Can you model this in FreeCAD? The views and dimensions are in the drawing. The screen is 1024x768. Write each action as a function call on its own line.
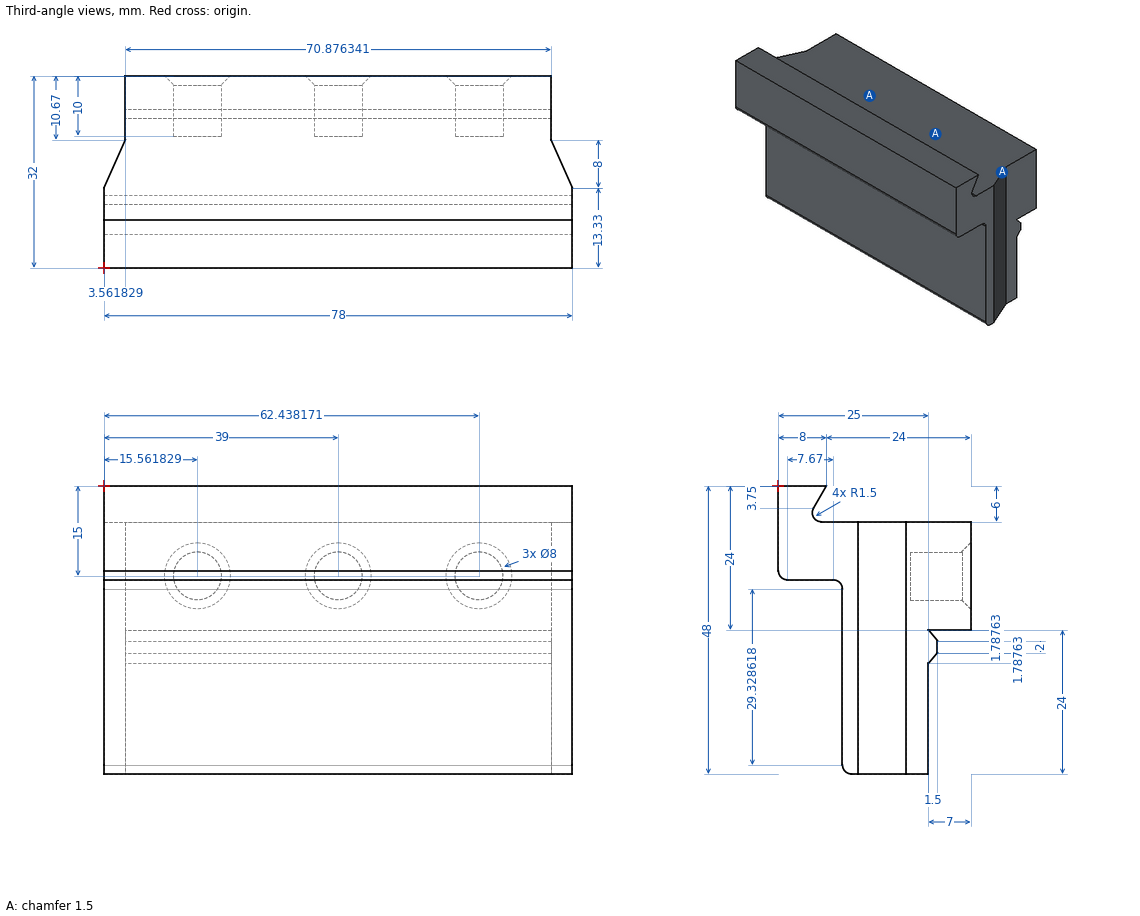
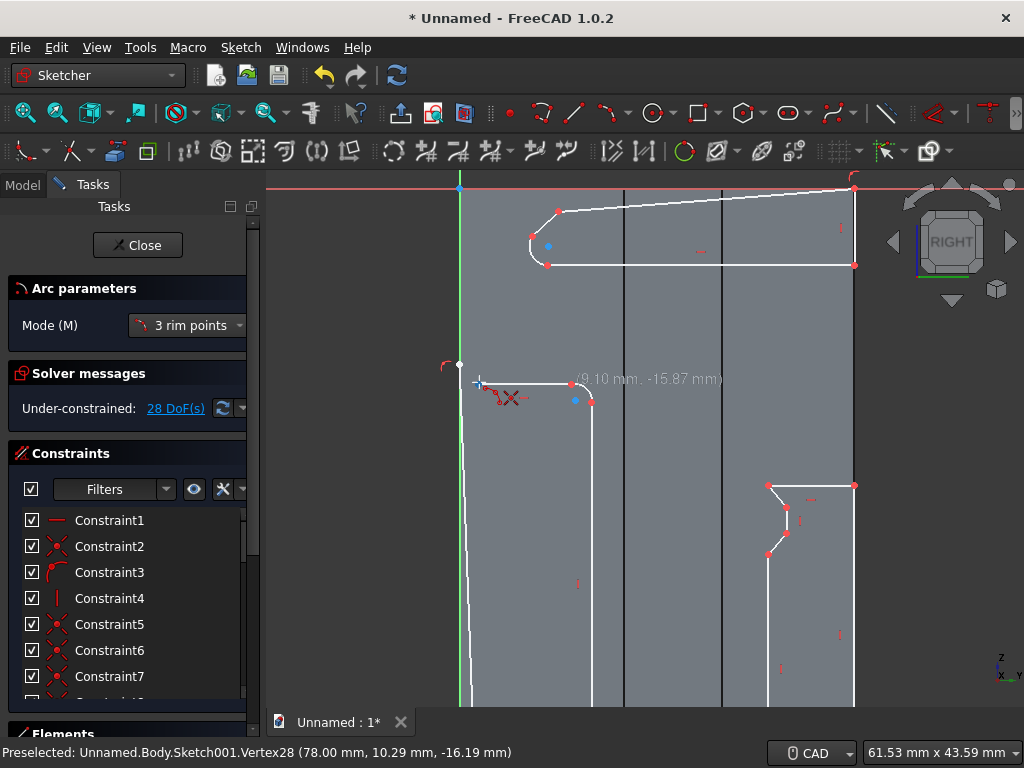
click(478, 384)
click(460, 365)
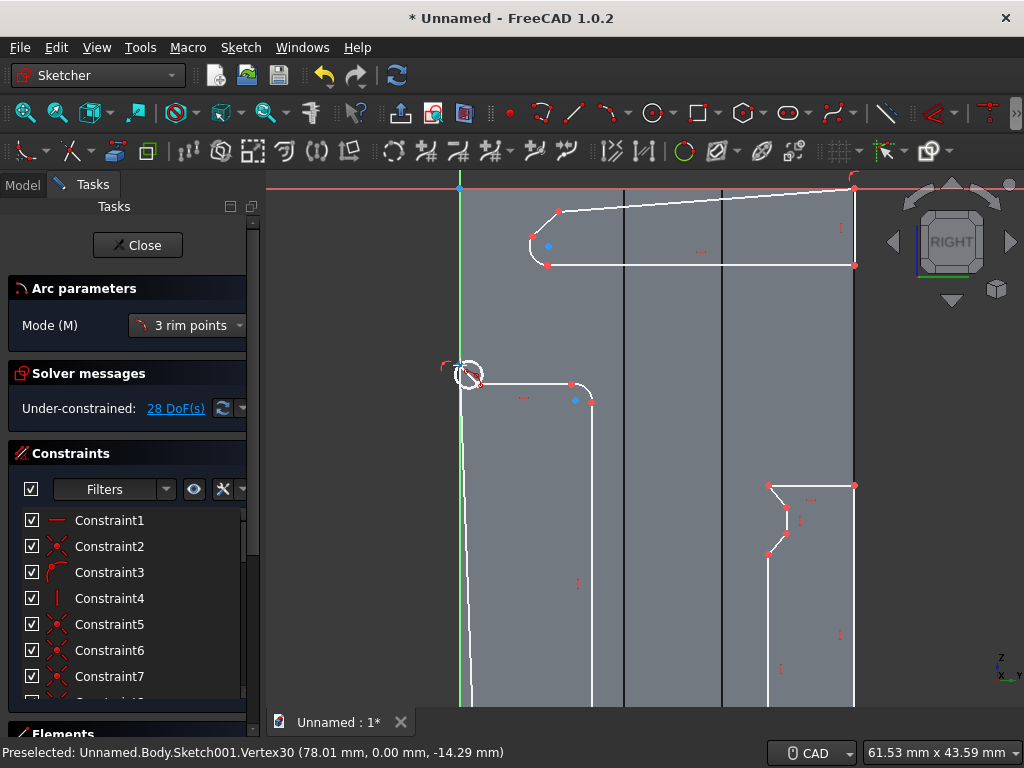
scroll(465, 377, up, 6)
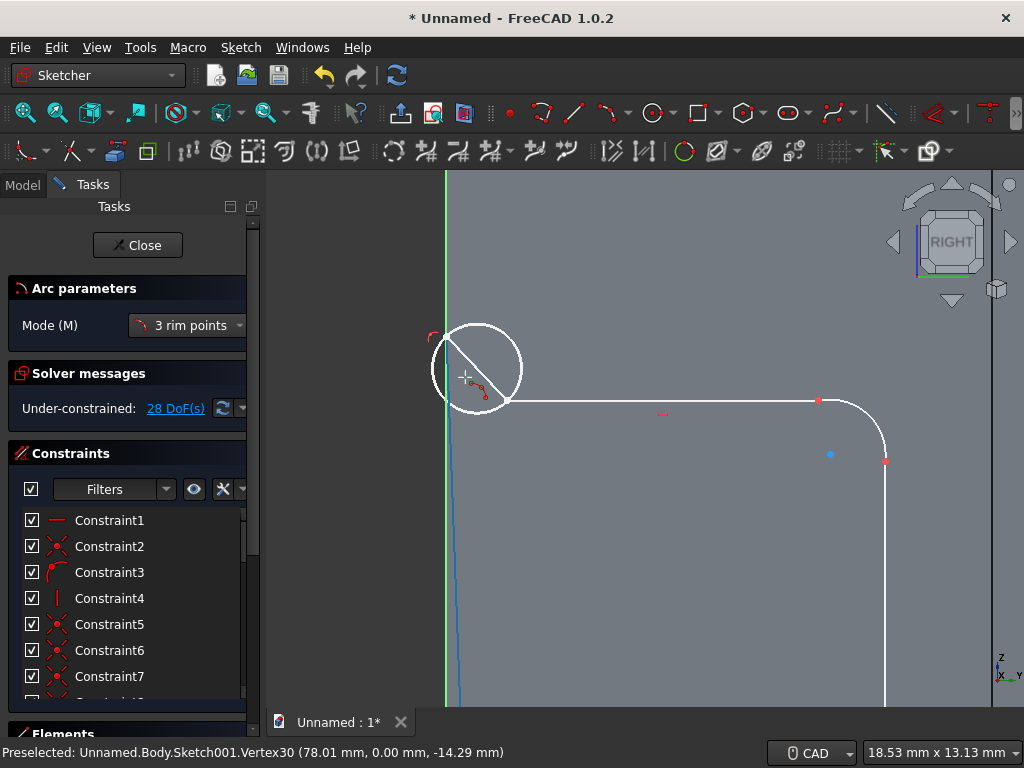
click(464, 375)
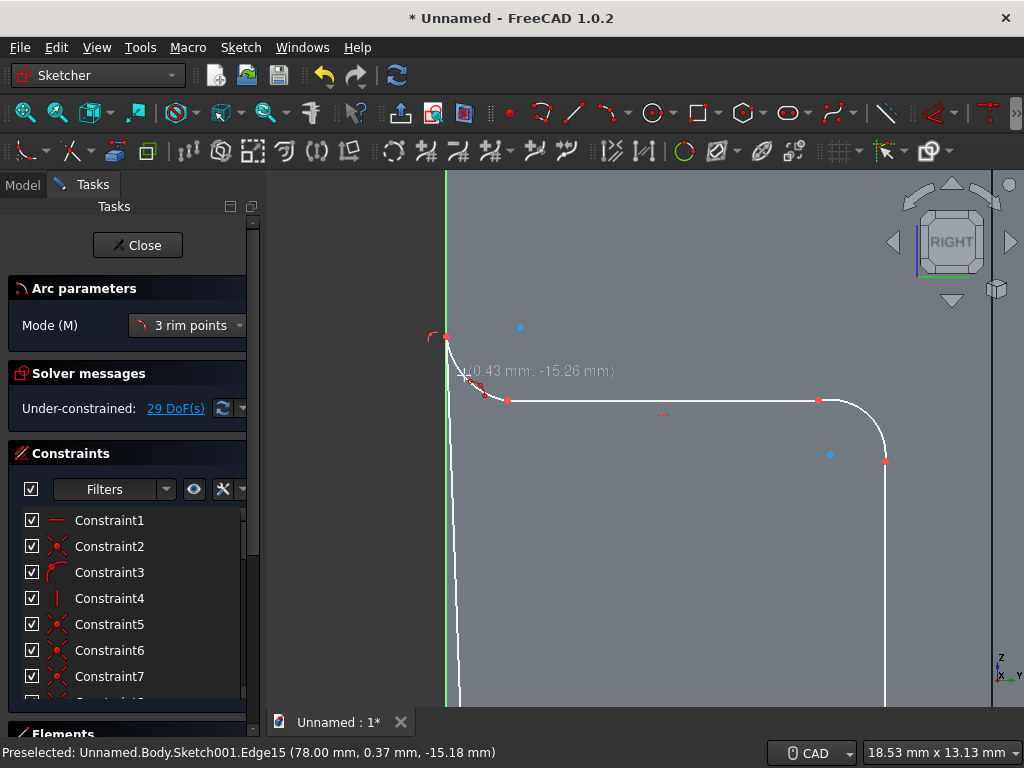
scroll(473, 380, down, 9)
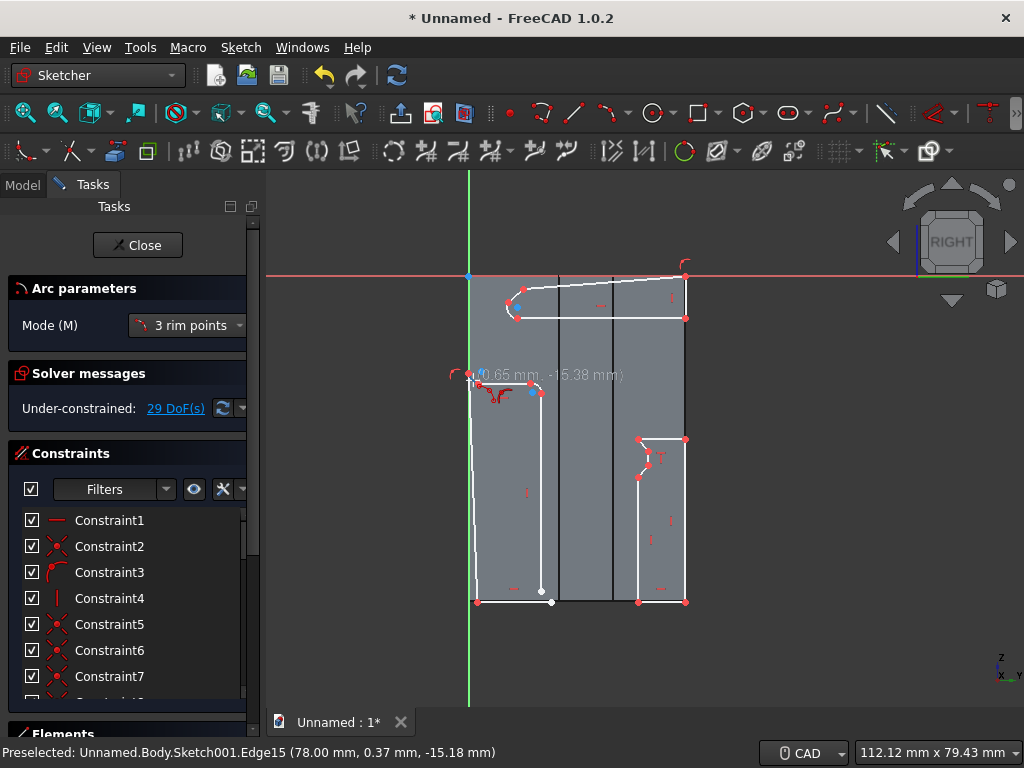
click(551, 602)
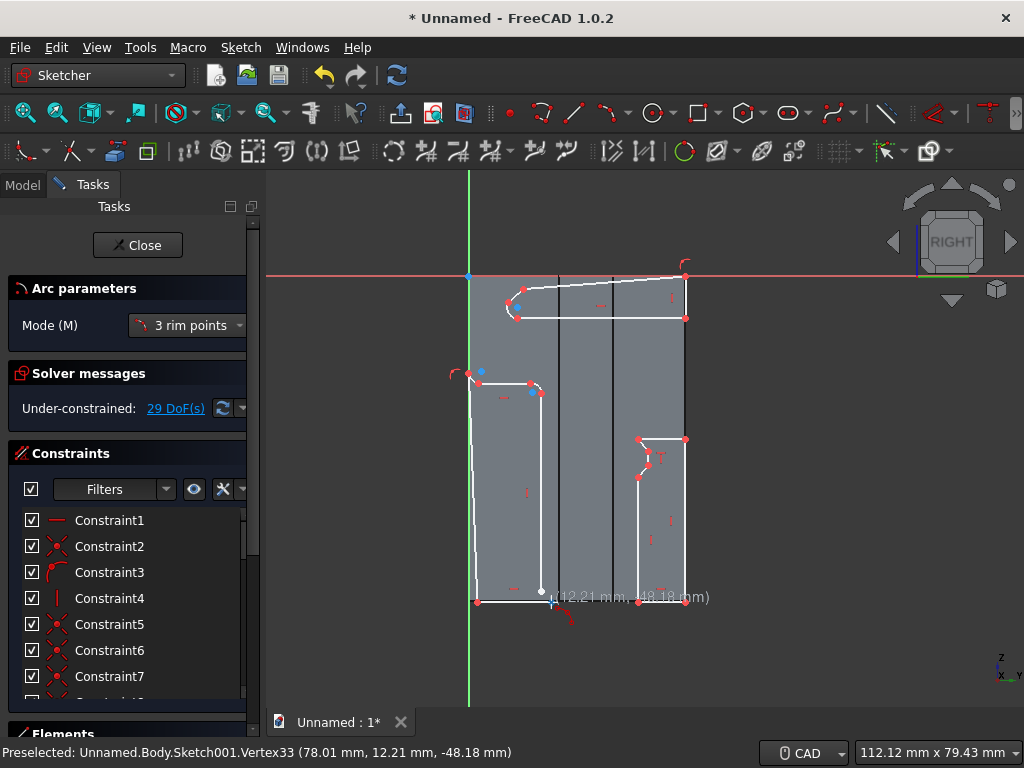
scroll(541, 591, up, 3)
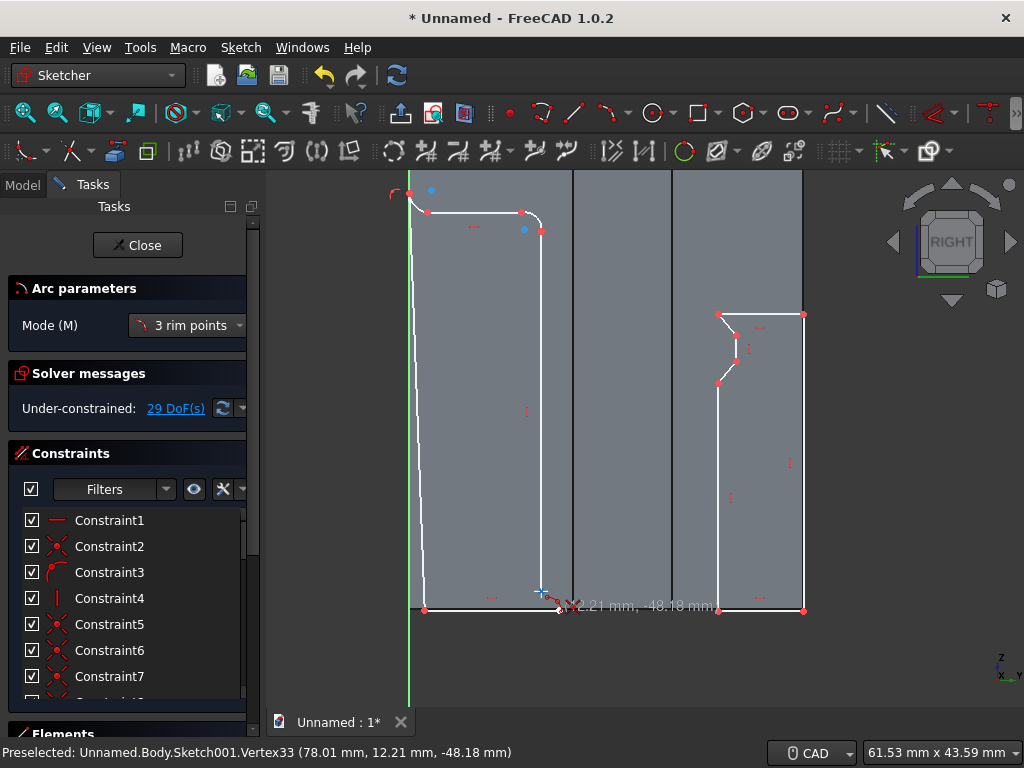
click(541, 592)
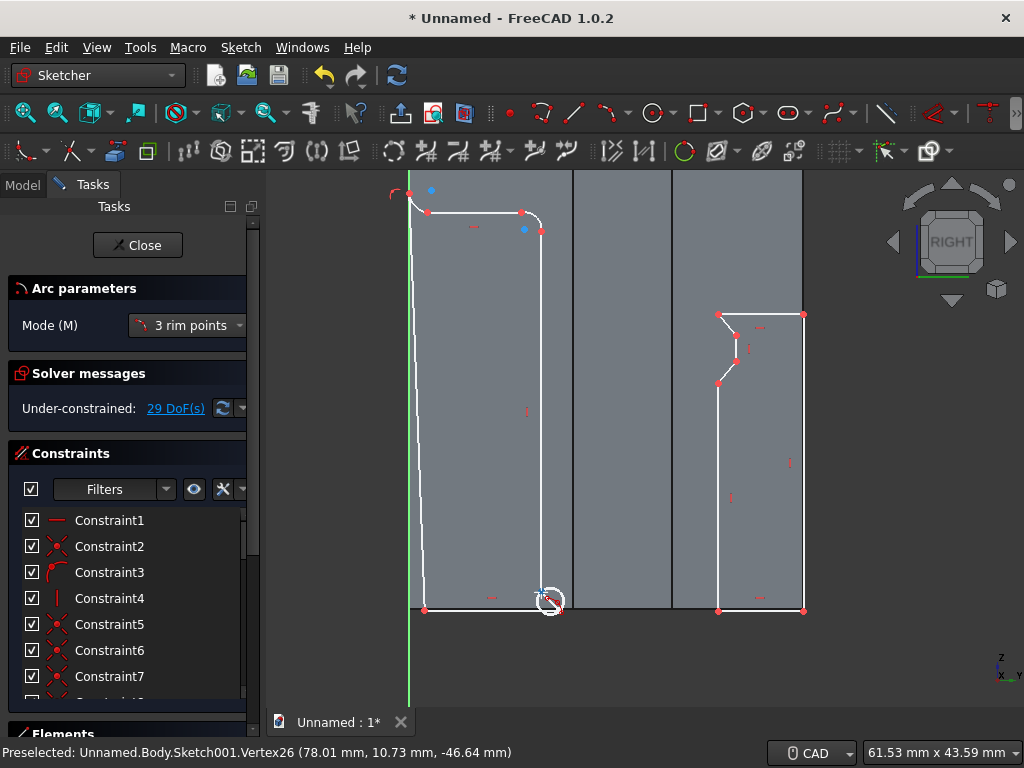
scroll(546, 603, up, 6)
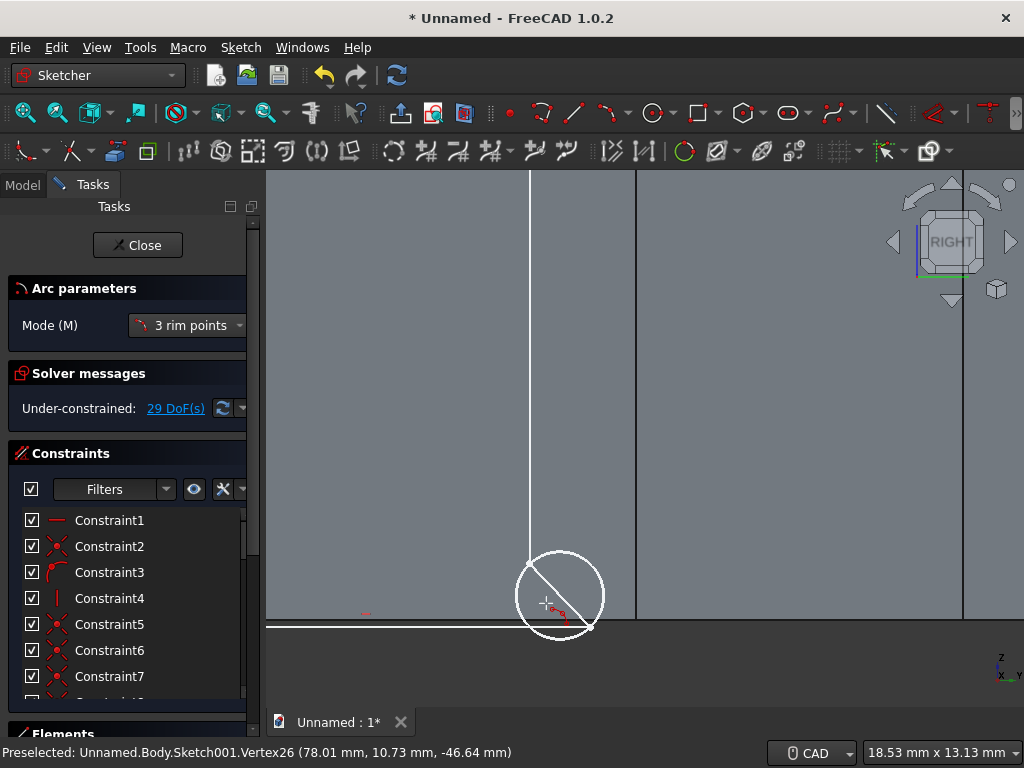
click(545, 602)
key(Escape)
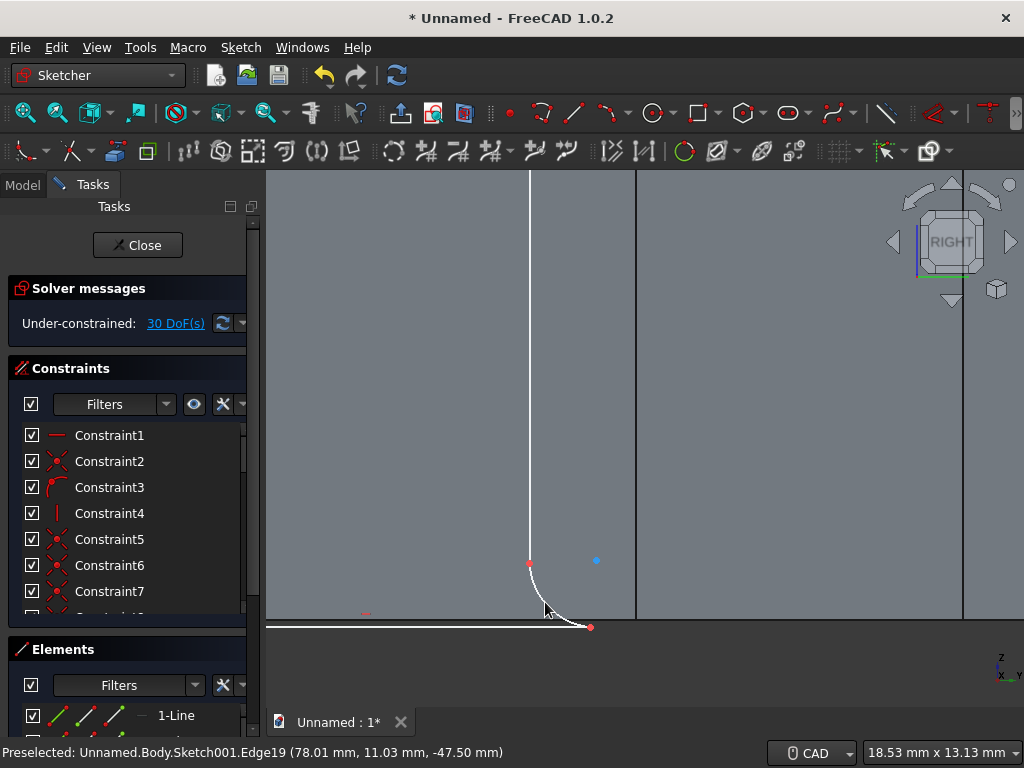
scroll(543, 597, down, 9)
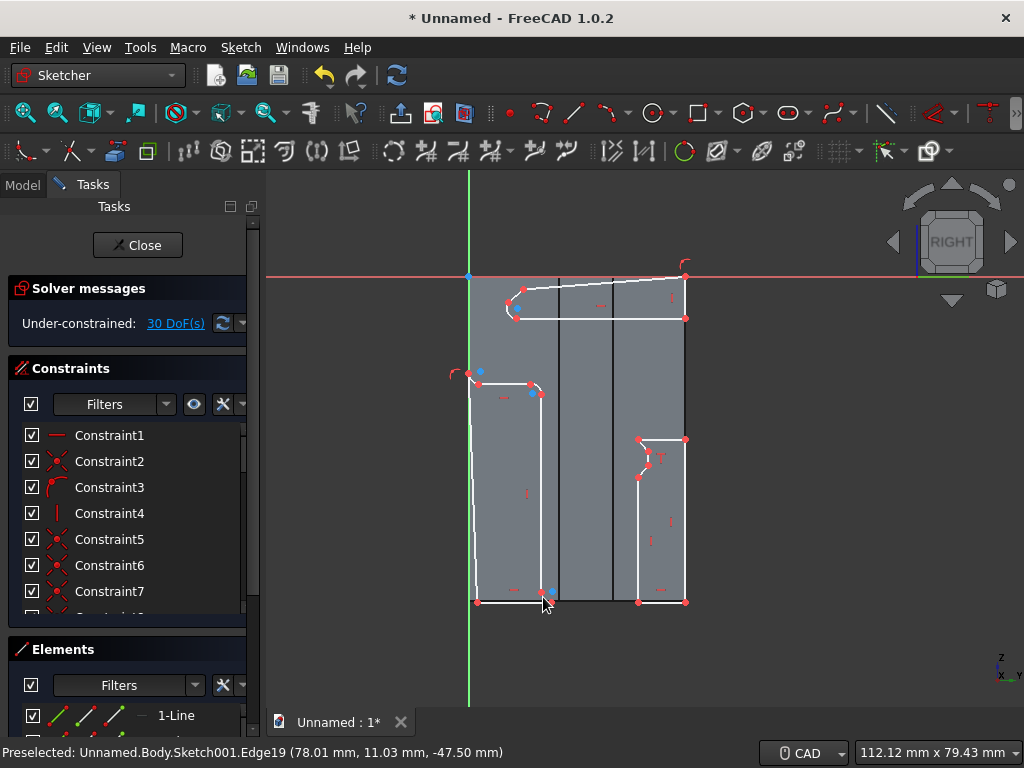
click(567, 319)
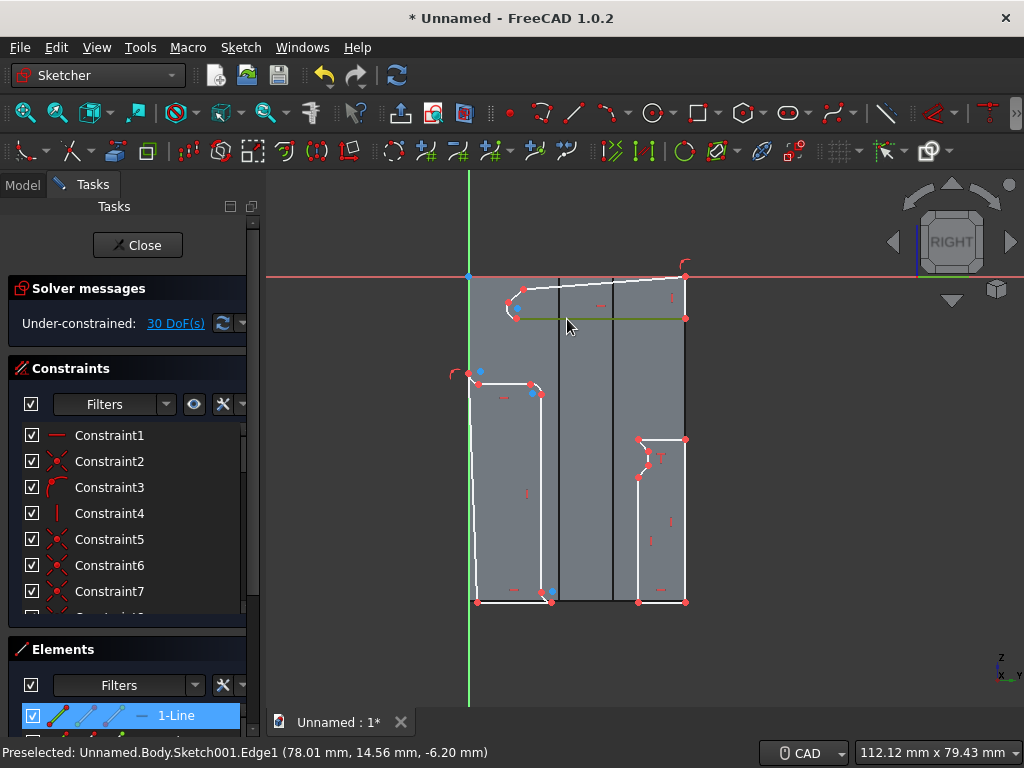
scroll(508, 313, up, 2)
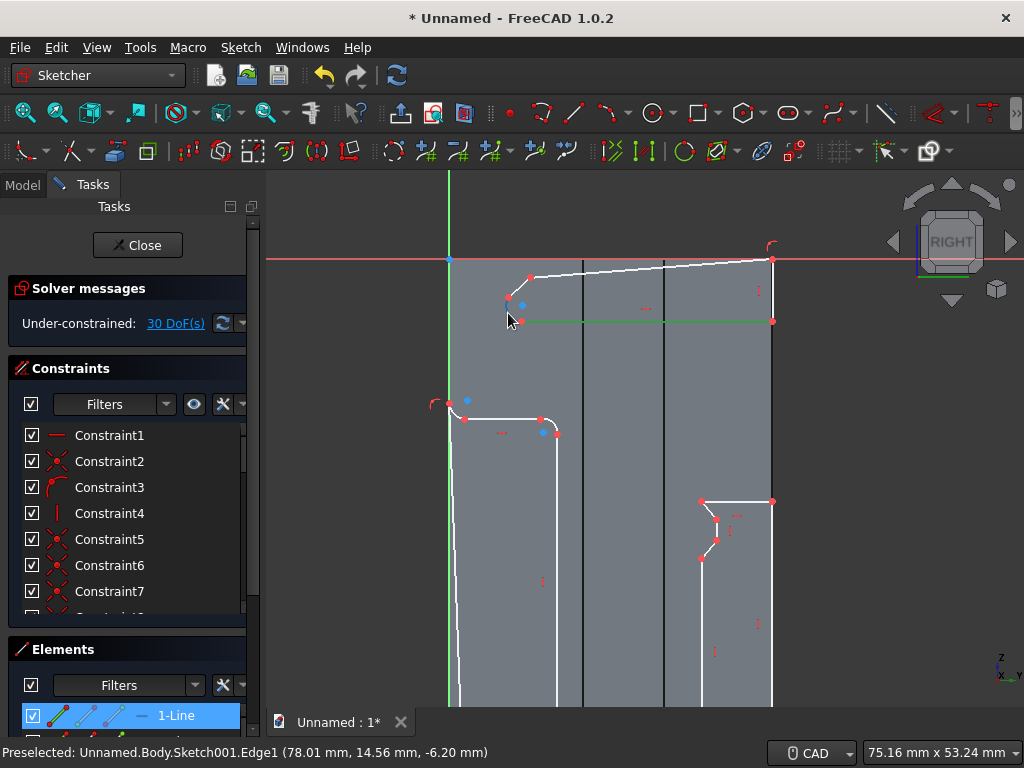
click(508, 313)